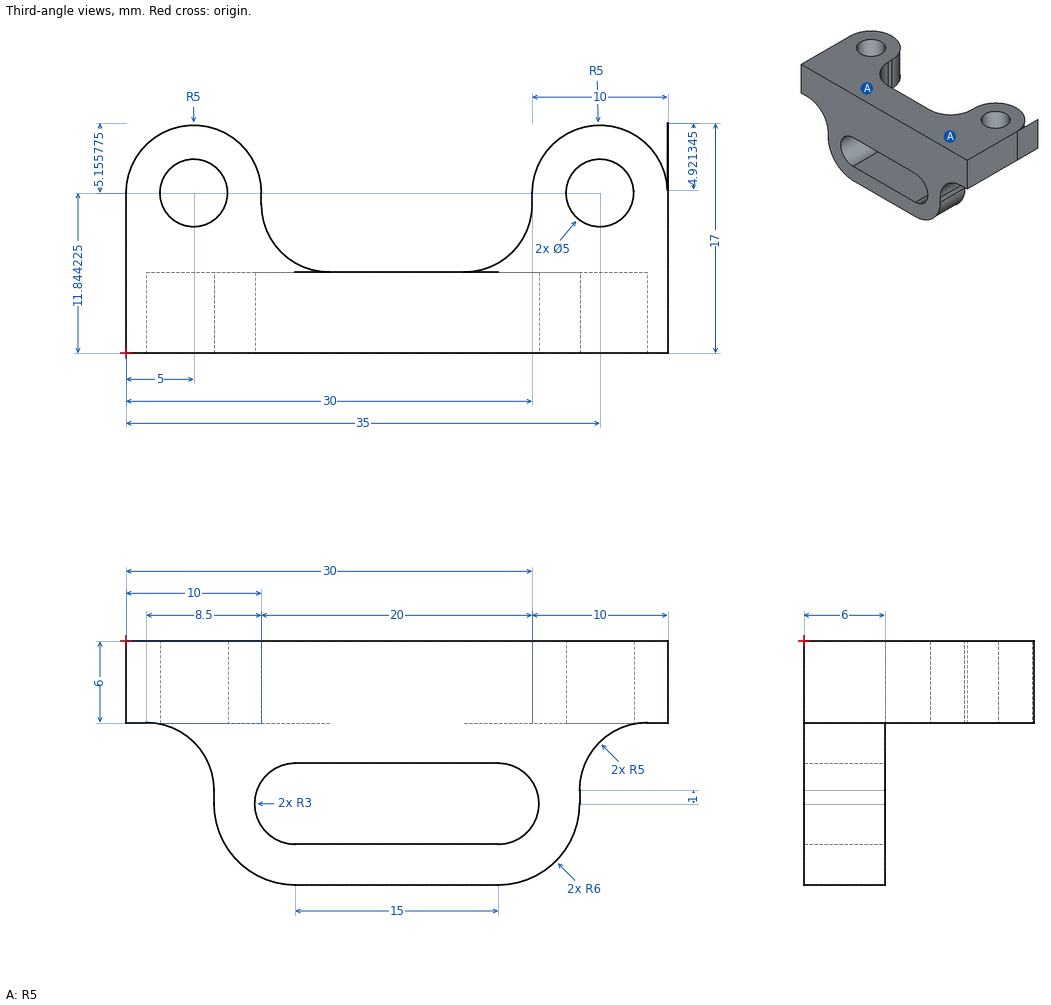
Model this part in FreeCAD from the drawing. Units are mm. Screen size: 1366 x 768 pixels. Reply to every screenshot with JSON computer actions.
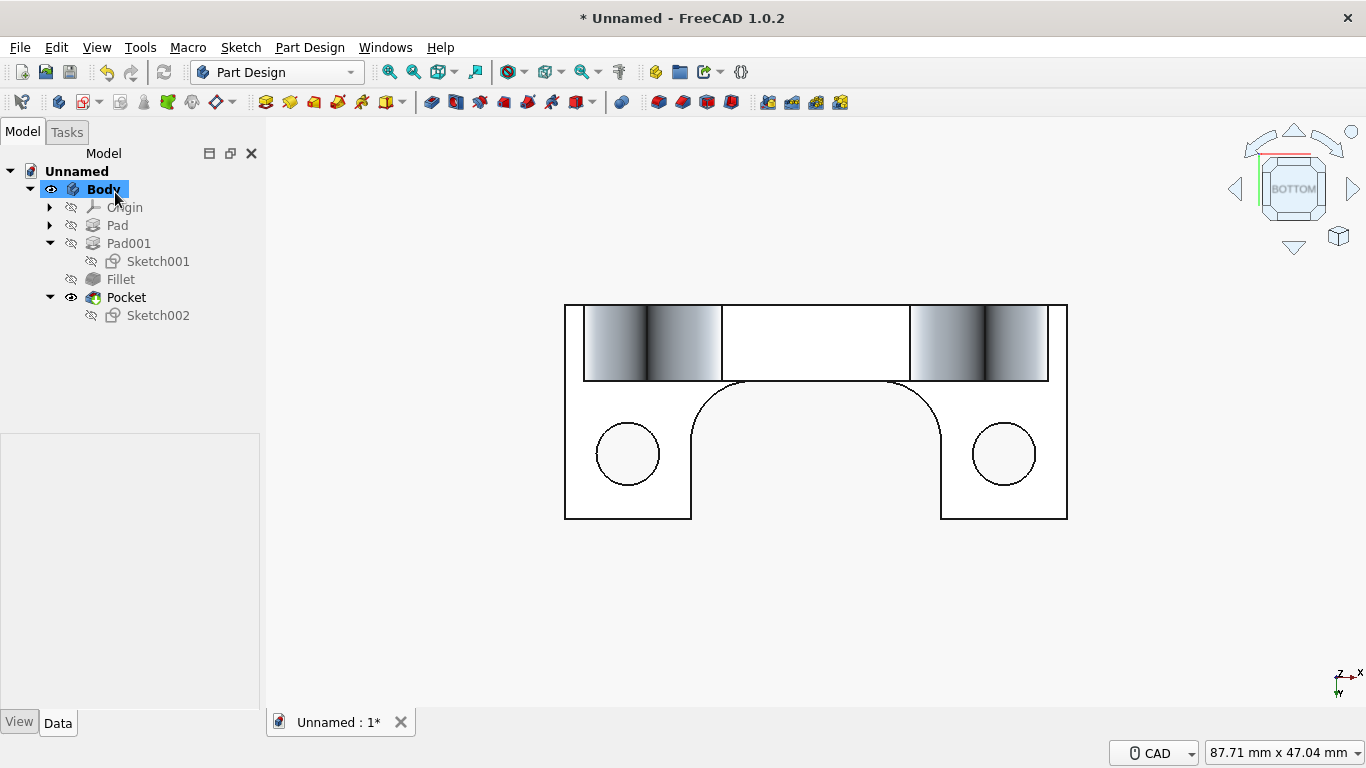
{"action": "left_click", "coordinate": [659, 411]}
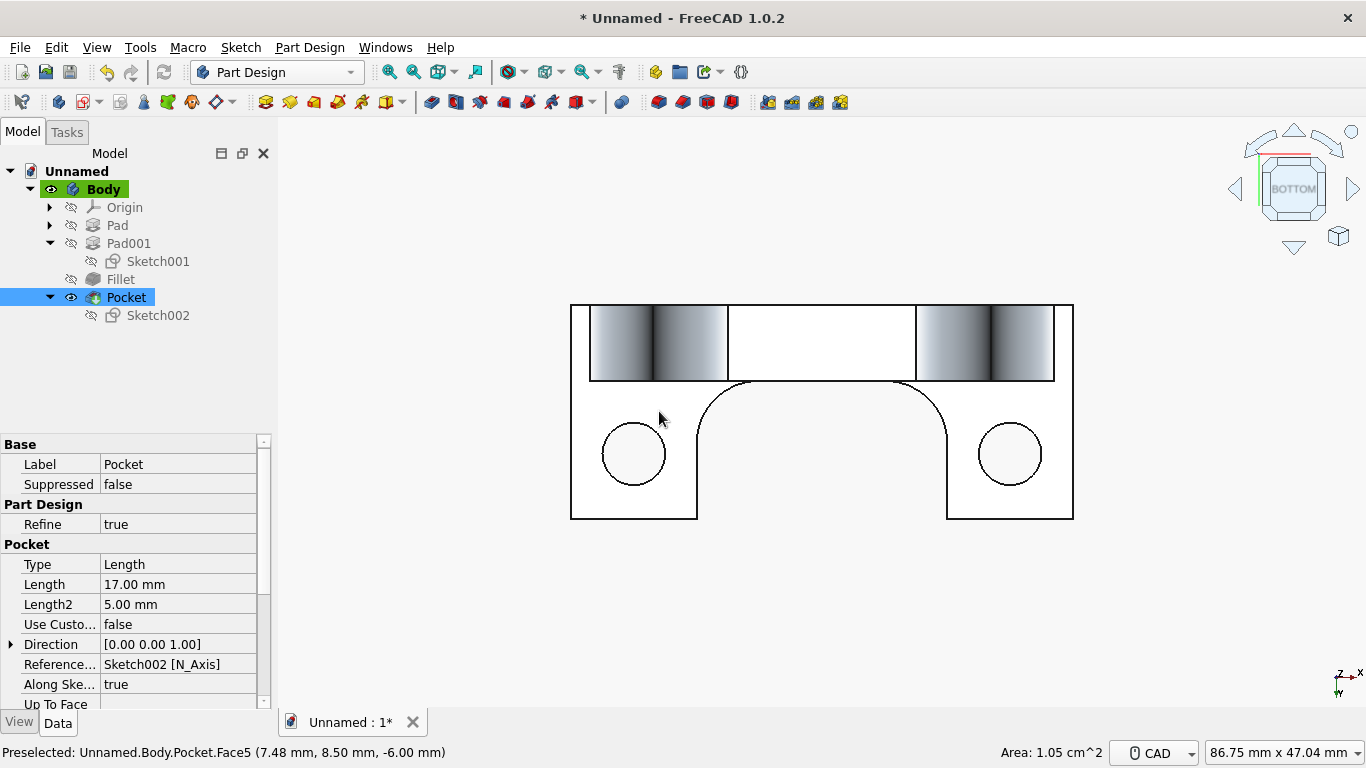
{"action": "left_click", "coordinate": [84, 102]}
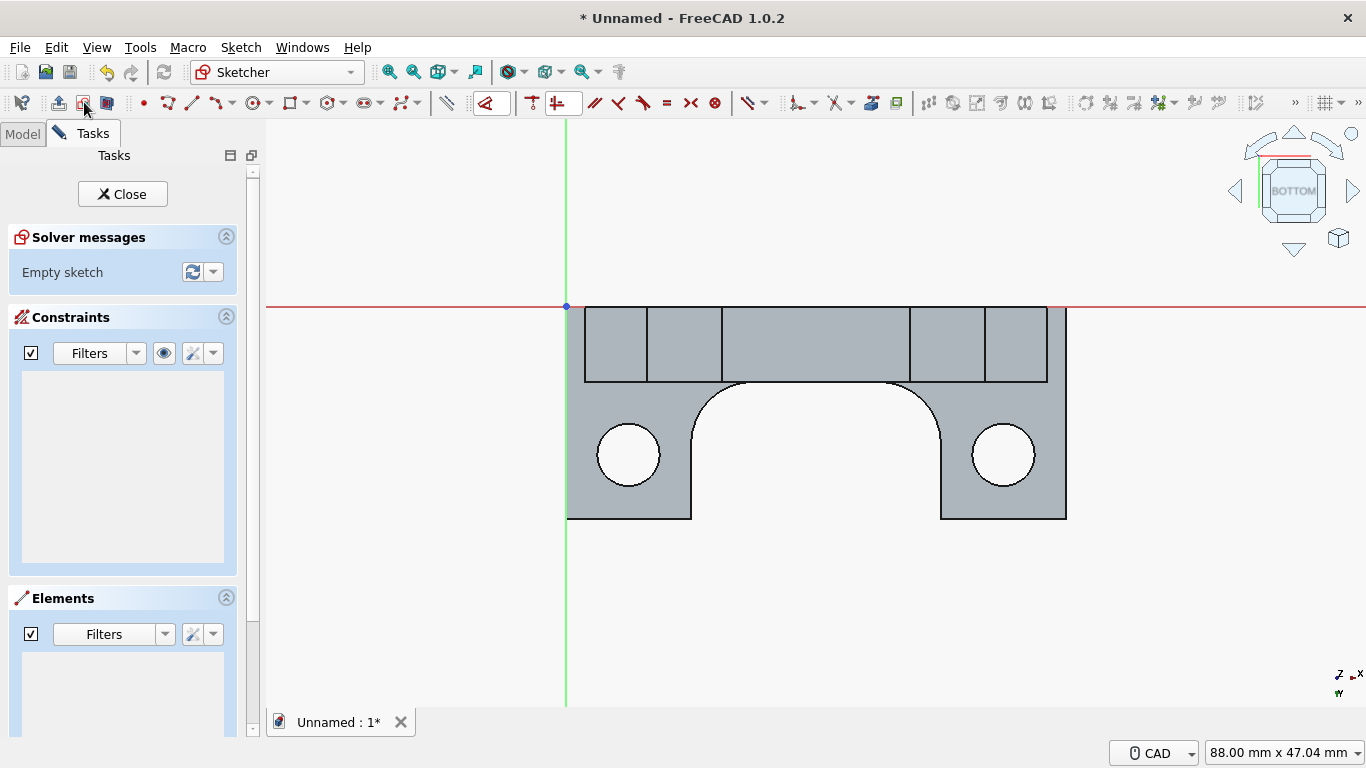
{"action": "key", "text": "q s"}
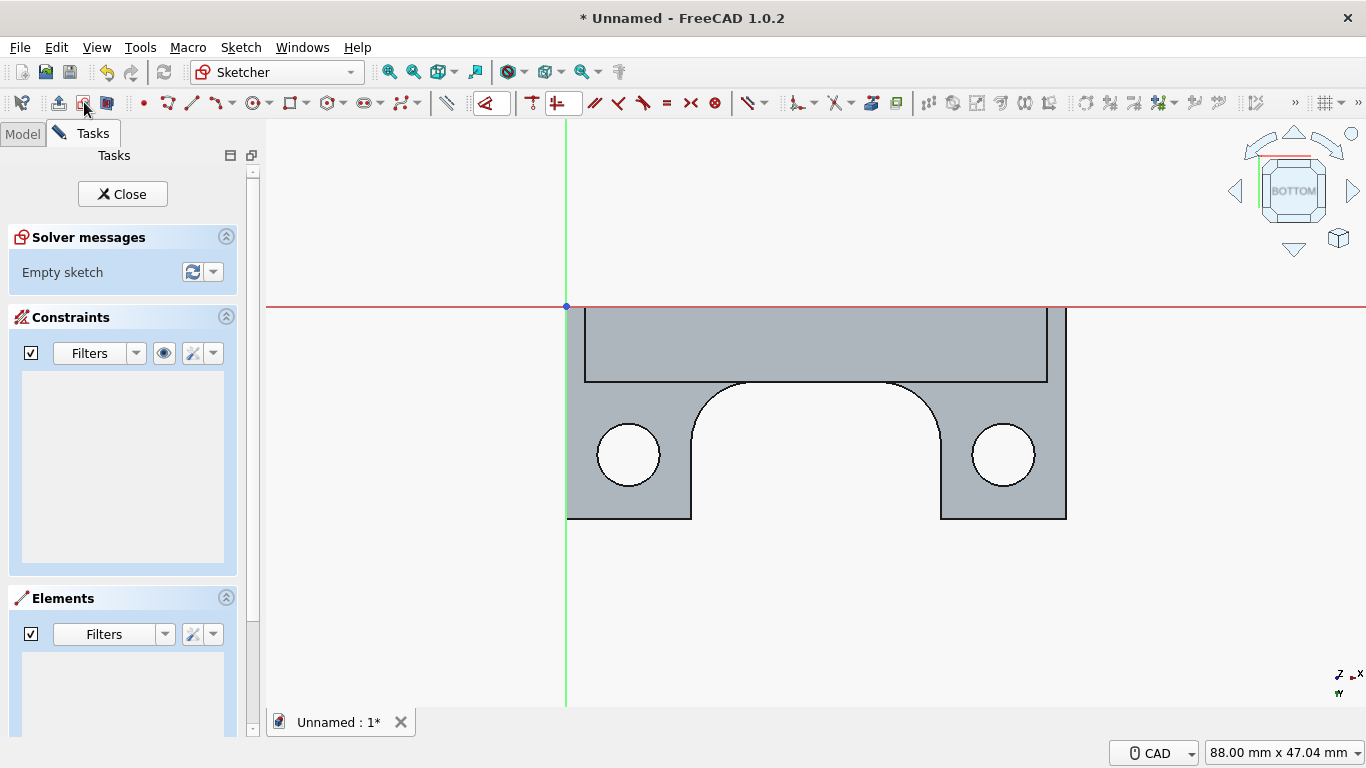
{"action": "scroll", "coordinate": [484, 413], "scroll_direction": "up", "scroll_amount": 3}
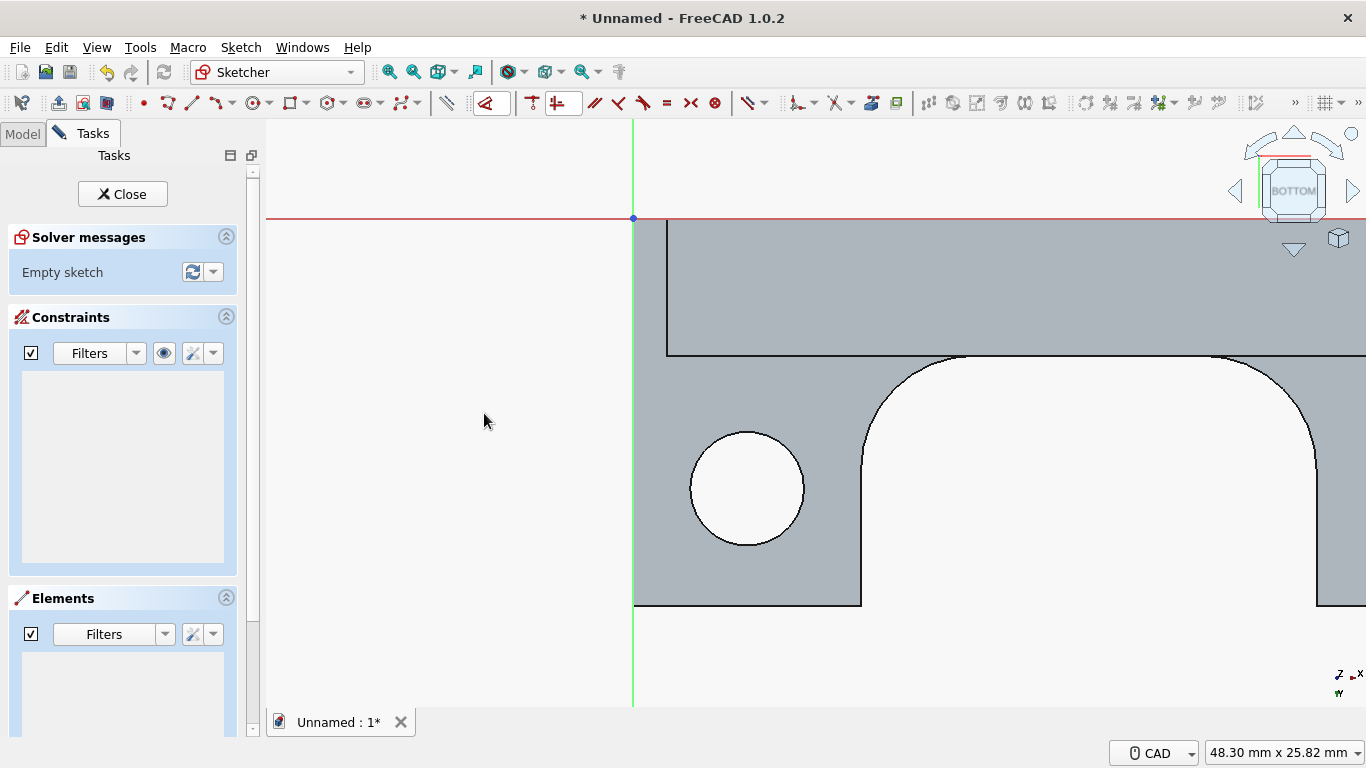
{"action": "left_click", "coordinate": [168, 104]}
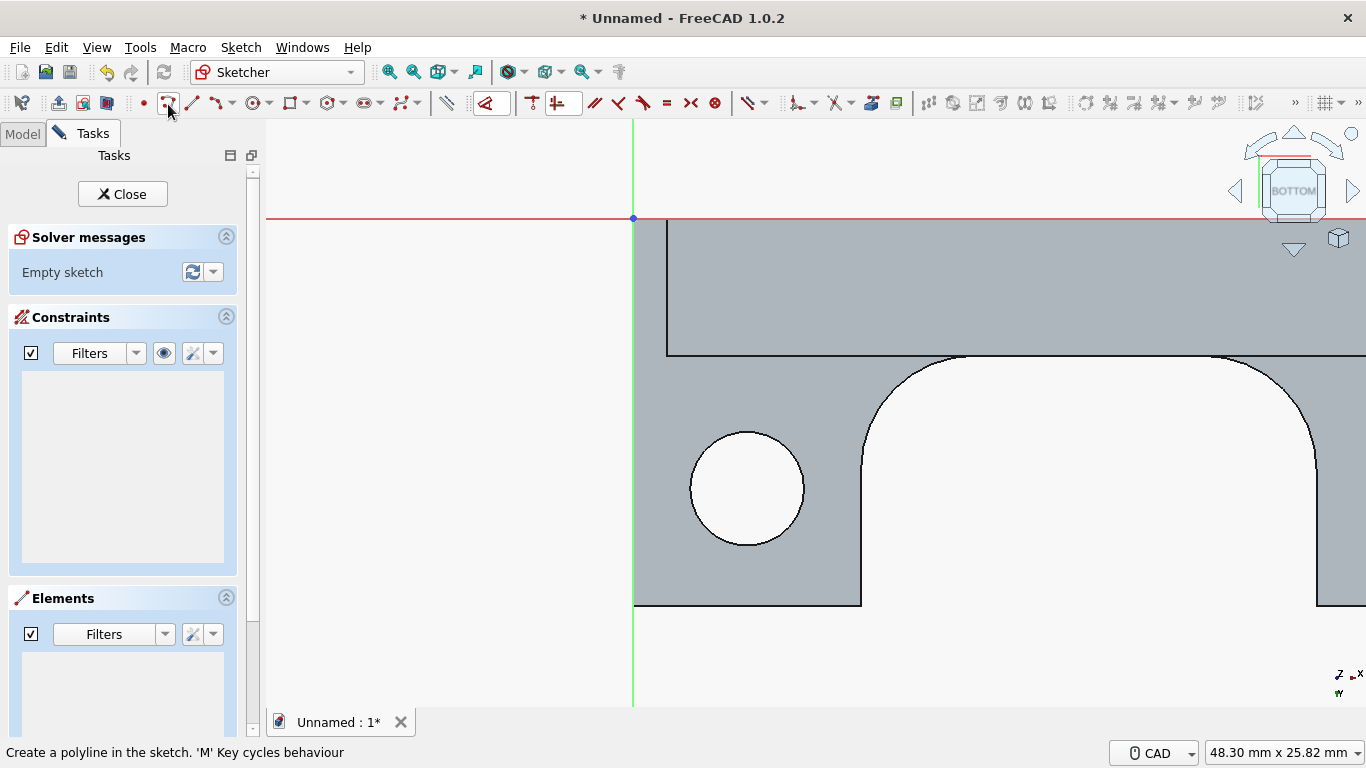
{"action": "left_click", "coordinate": [633, 489]}
{"action": "left_click", "coordinate": [642, 606]}
{"action": "left_click", "coordinate": [861, 606]}
{"action": "left_click", "coordinate": [861, 489]}
{"action": "right_click", "coordinate": [861, 489]}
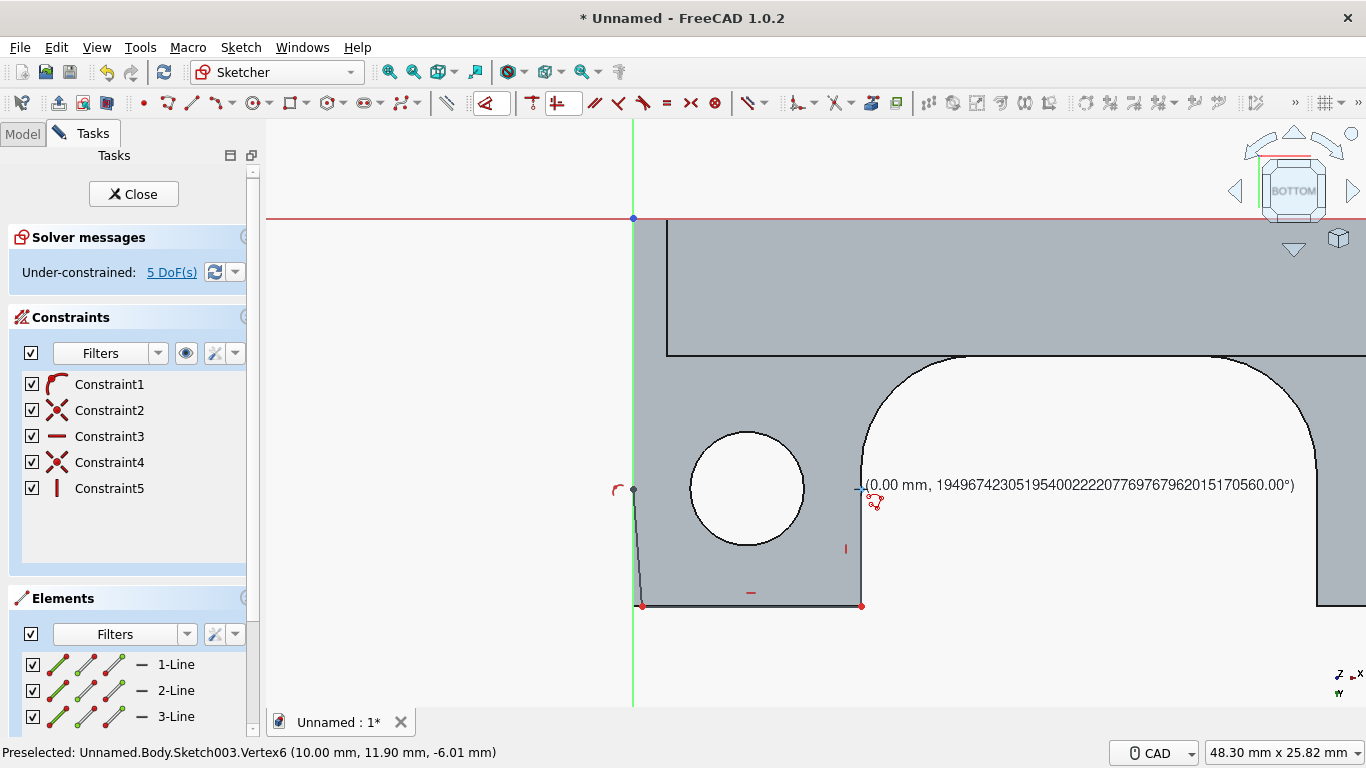
{"action": "left_click", "coordinate": [216, 104]}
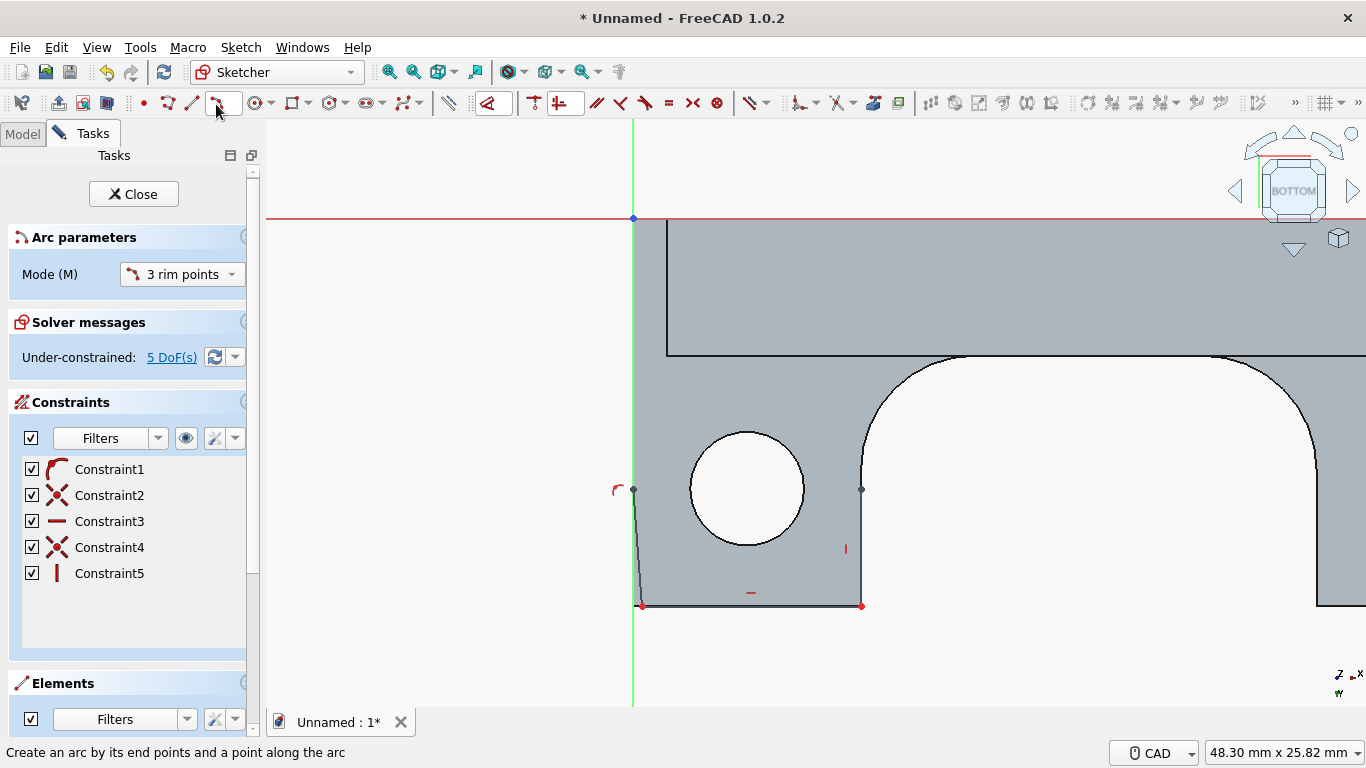
{"action": "left_click", "coordinate": [861, 490]}
{"action": "left_click", "coordinate": [633, 490]}
{"action": "left_click", "coordinate": [680, 581]}
{"action": "key", "text": "Escape"}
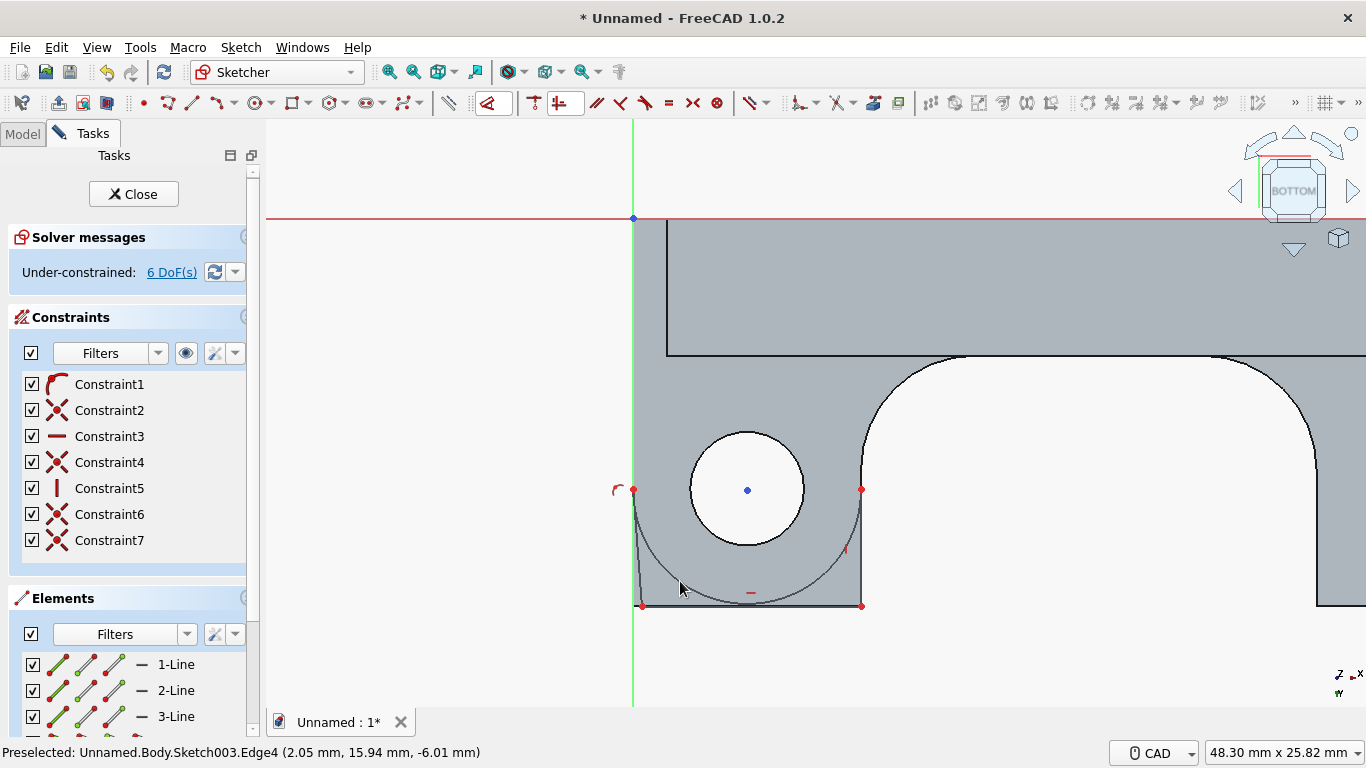
{"action": "scroll", "coordinate": [640, 584], "scroll_direction": "up", "scroll_amount": 4}